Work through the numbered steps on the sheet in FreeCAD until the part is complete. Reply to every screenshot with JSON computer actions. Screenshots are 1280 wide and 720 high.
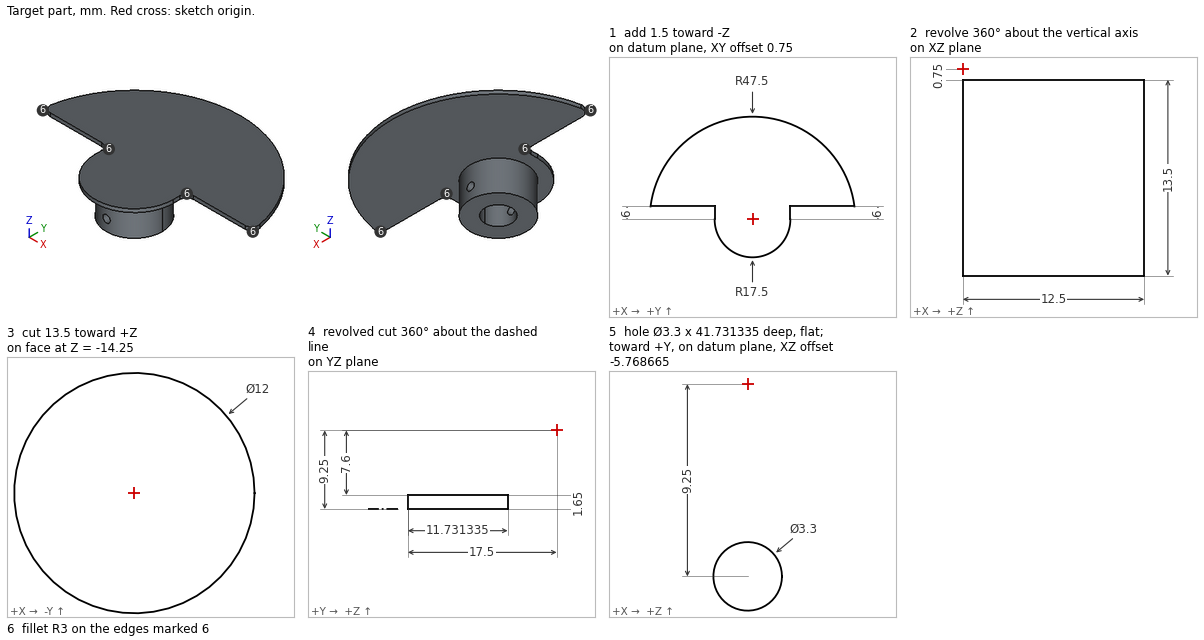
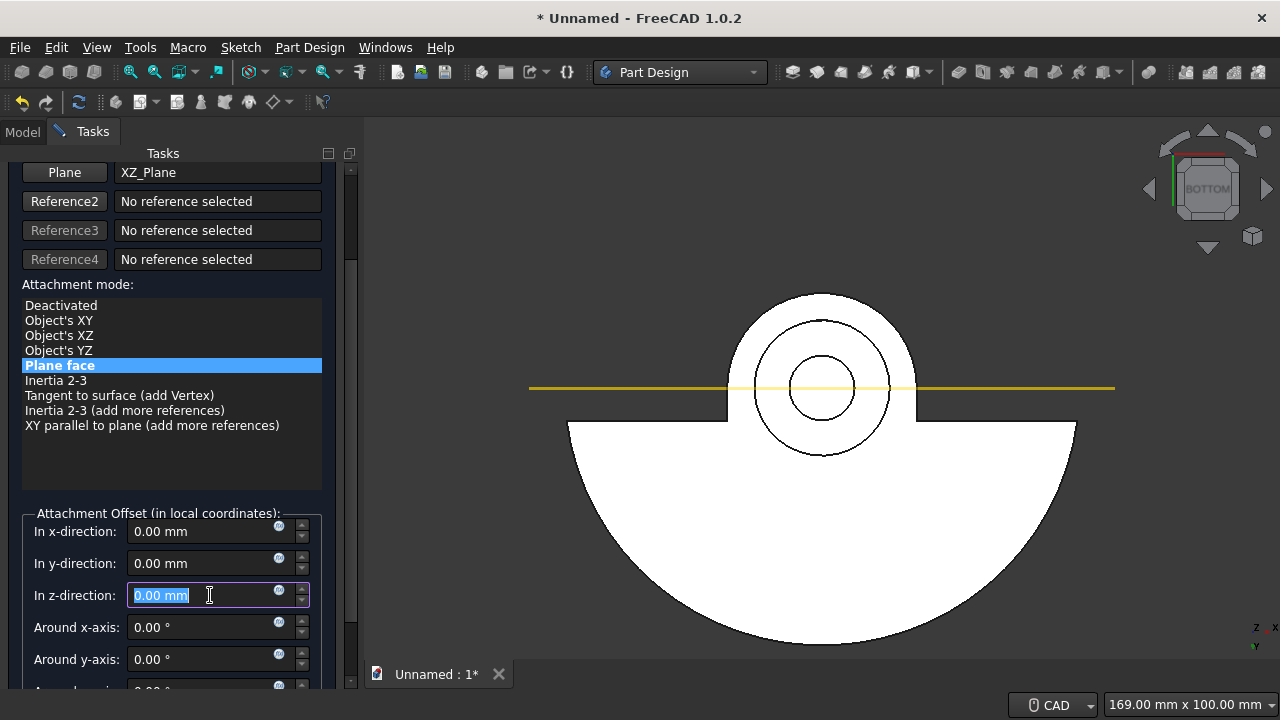
{"action": "type", "text": "-5.768665"}
{"action": "key", "text": "Tab"}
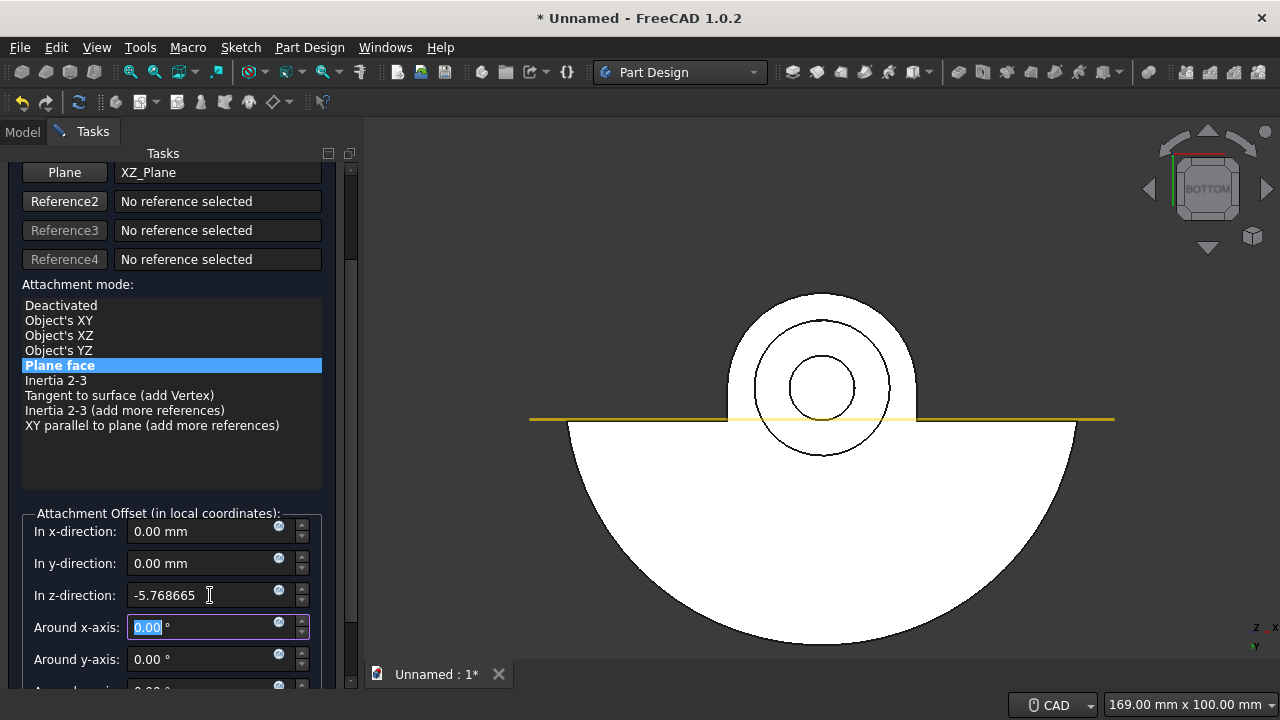
{"action": "scroll", "coordinate": [351, 426], "scroll_direction": "up", "scroll_amount": 3}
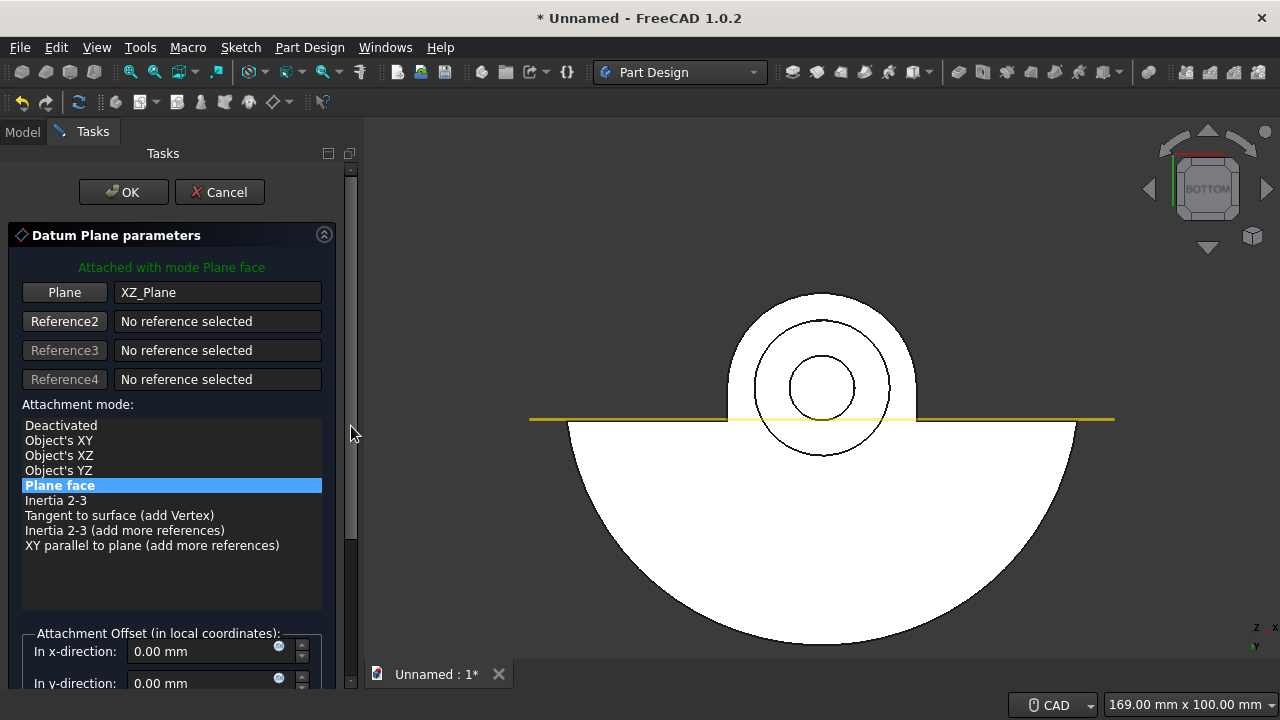
{"action": "left_click", "coordinate": [124, 192]}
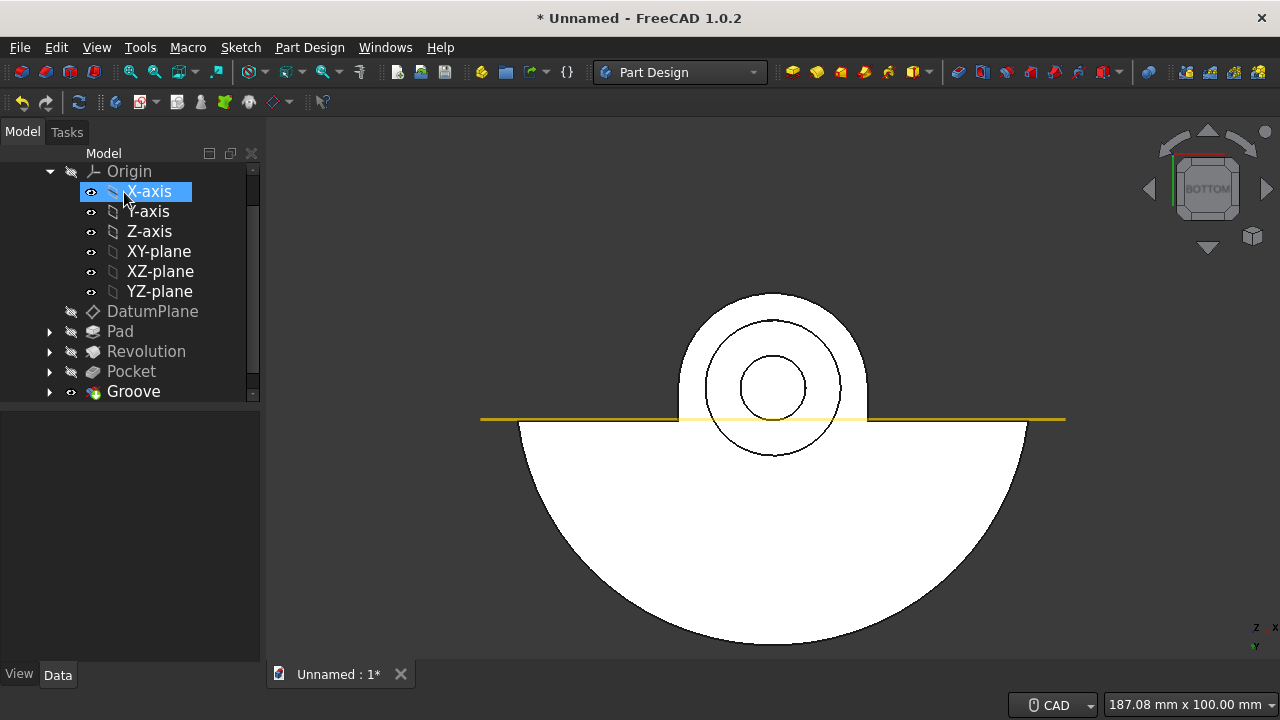
{"action": "scroll", "coordinate": [140, 287], "scroll_direction": "down", "scroll_amount": 3}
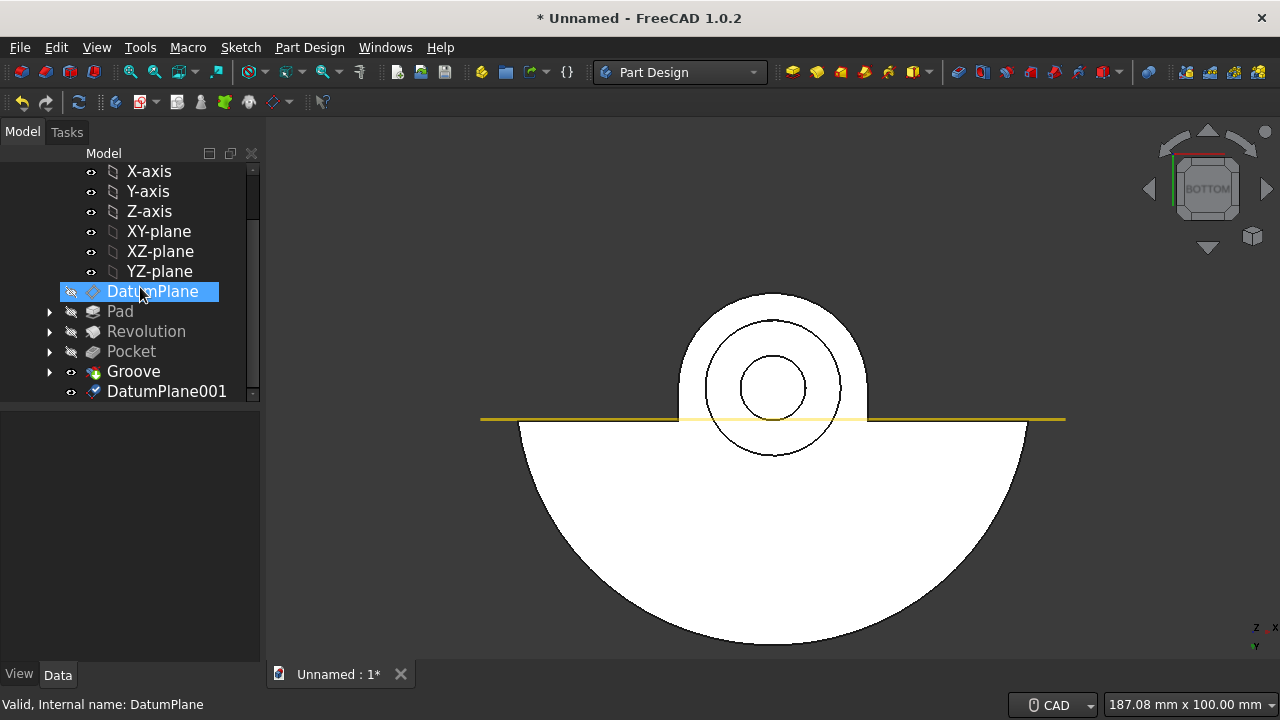
{"action": "left_click", "coordinate": [116, 392]}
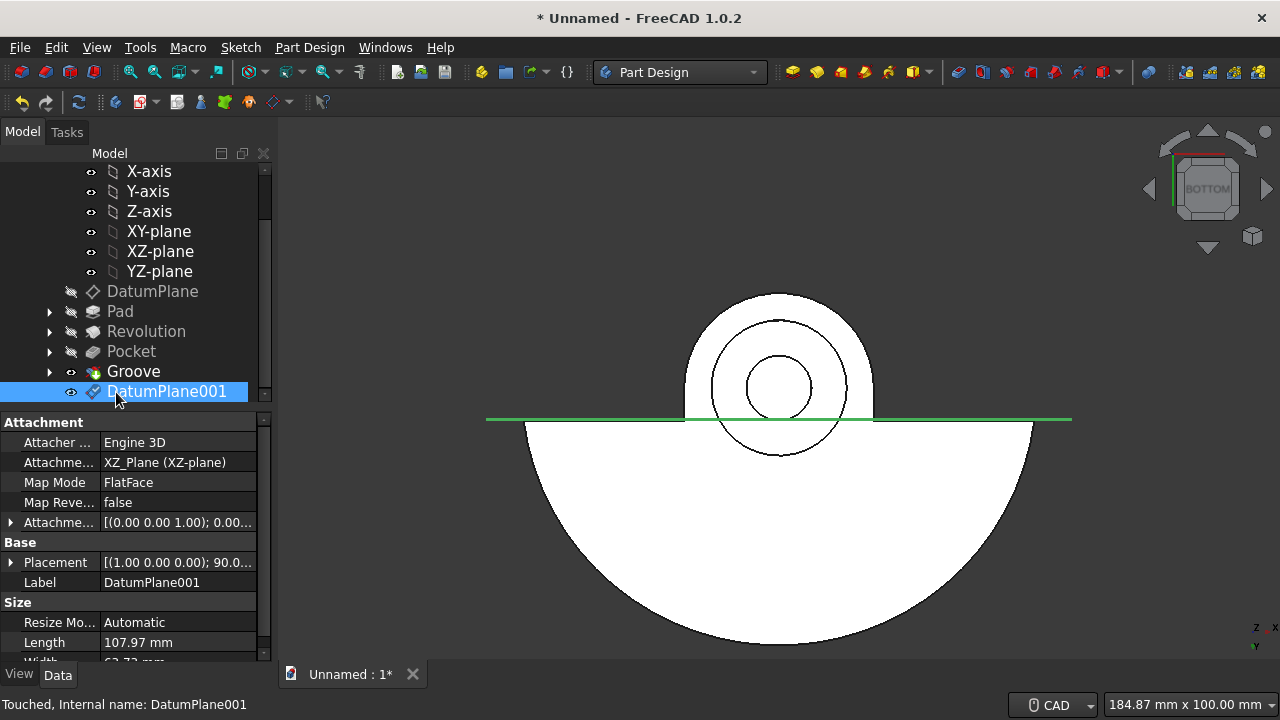
{"action": "left_click", "coordinate": [140, 102]}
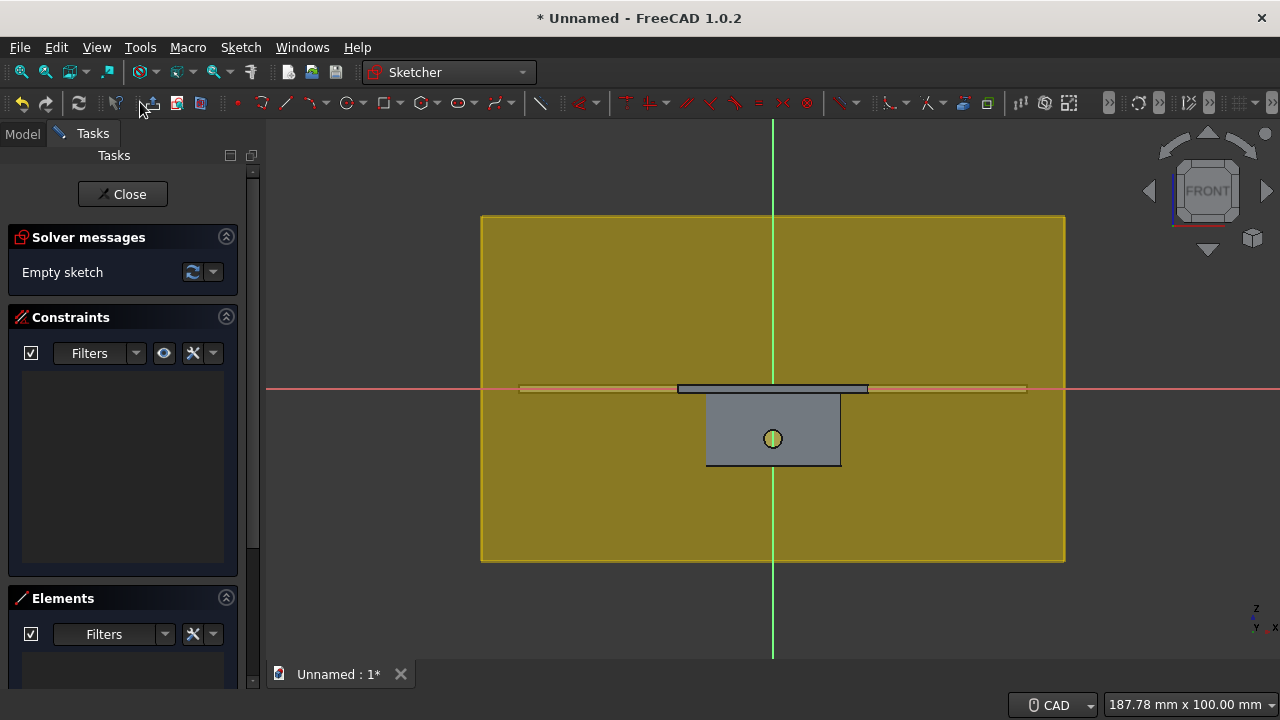
{"action": "key", "text": "q s"}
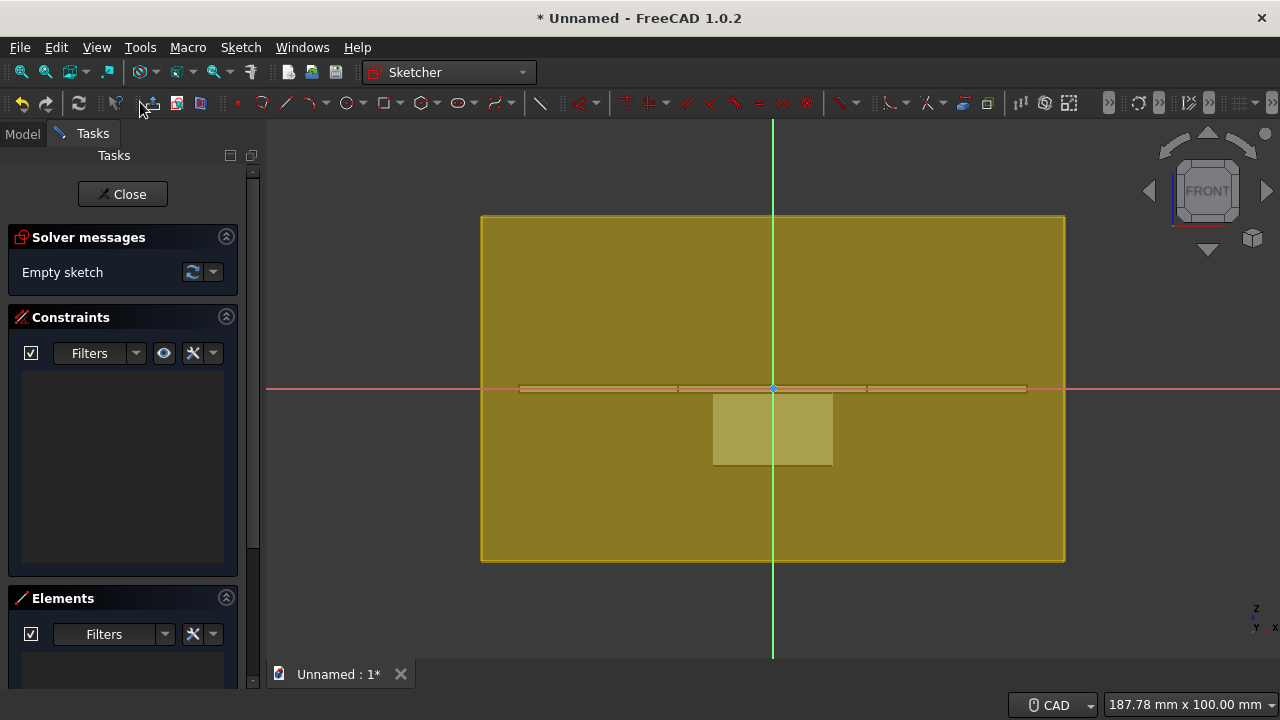
{"action": "scroll", "coordinate": [777, 442], "scroll_direction": "up", "scroll_amount": 15}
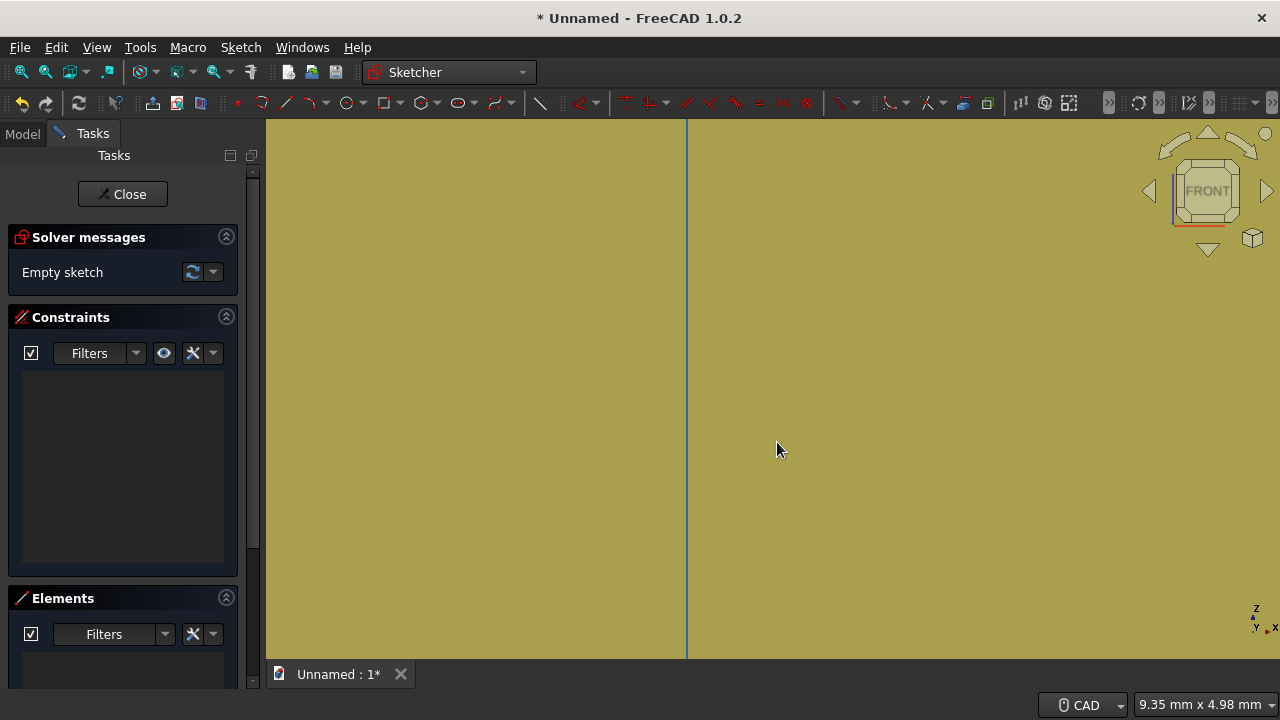
{"action": "key", "text": "g c"}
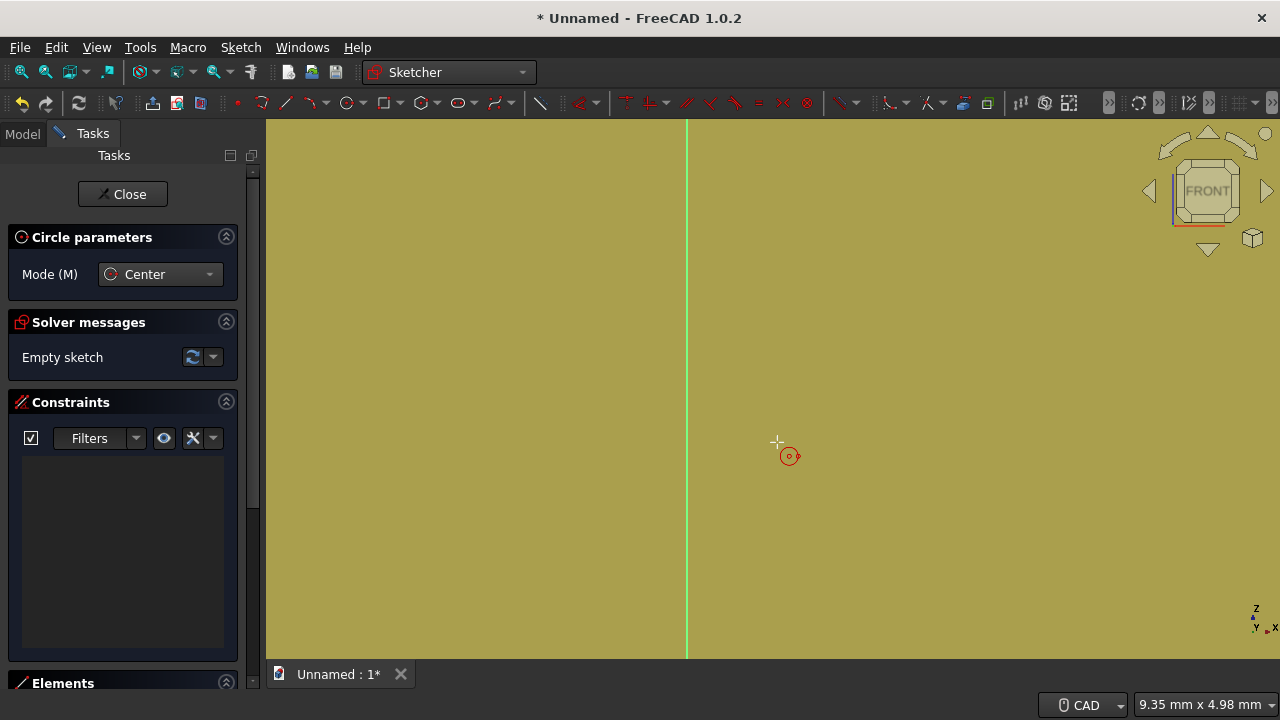
{"action": "left_click", "coordinate": [687, 369]}
{"action": "mouse_move", "coordinate": [814, 243]}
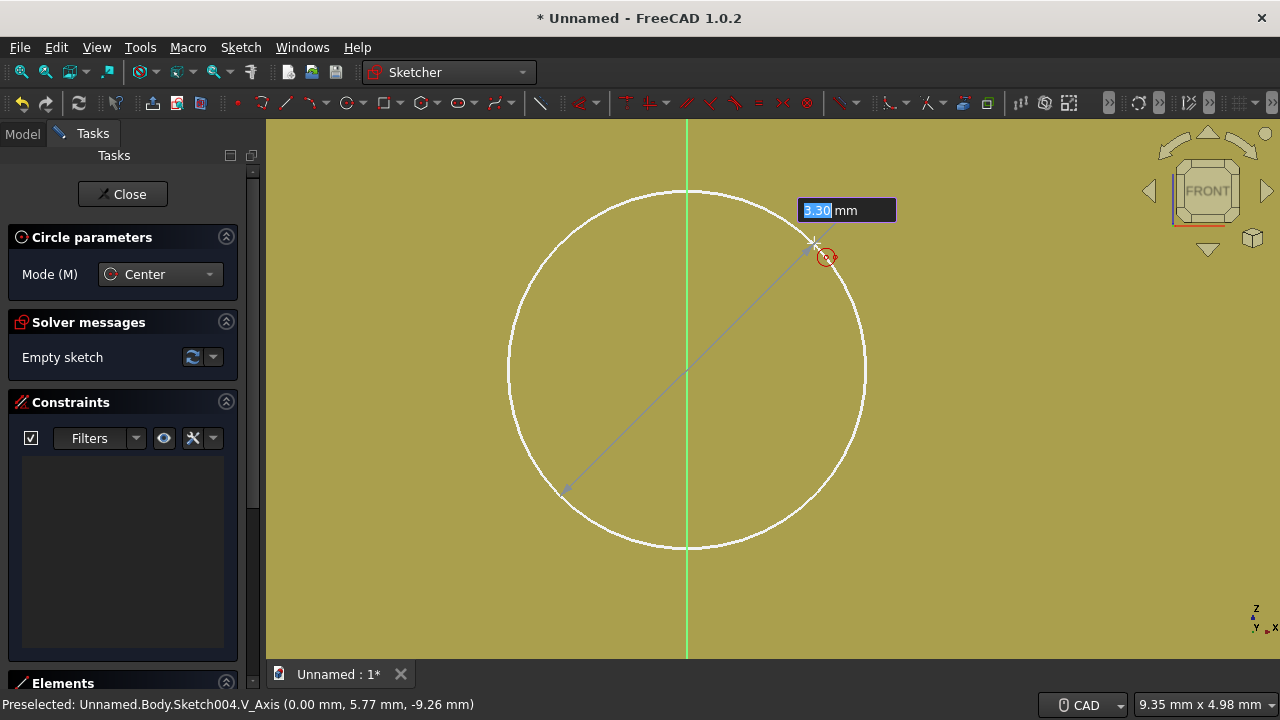
{"action": "type", "text": "3.3"}
{"action": "key", "text": "Return"}
{"action": "key", "text": "Escape"}